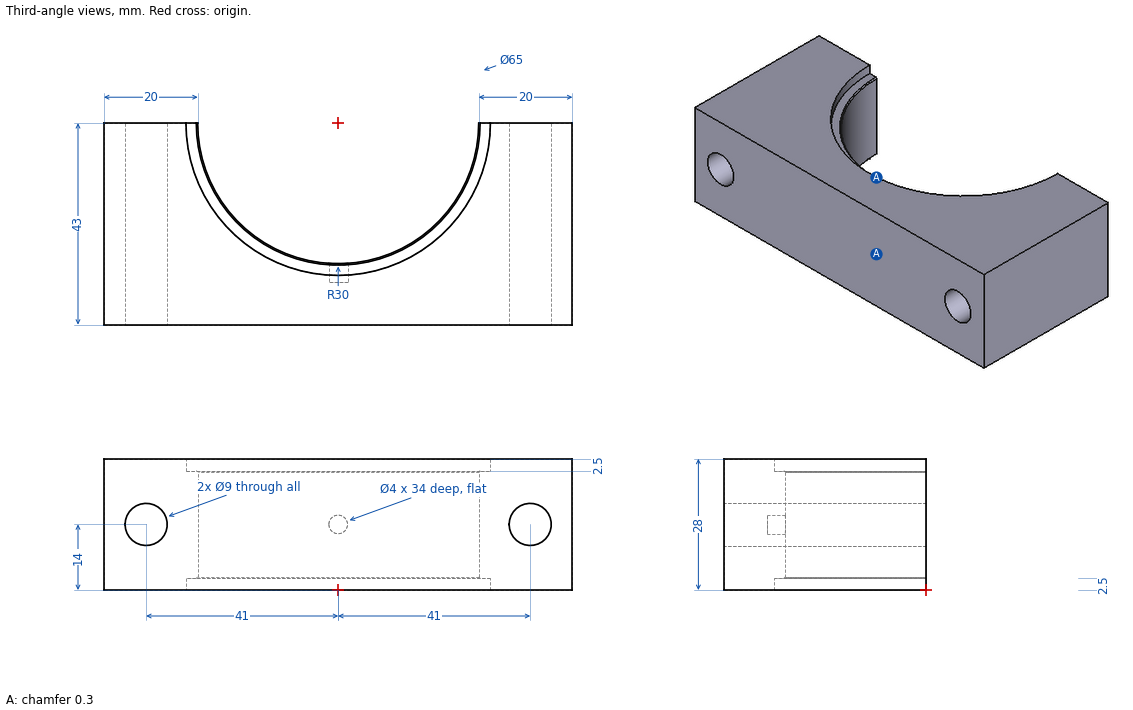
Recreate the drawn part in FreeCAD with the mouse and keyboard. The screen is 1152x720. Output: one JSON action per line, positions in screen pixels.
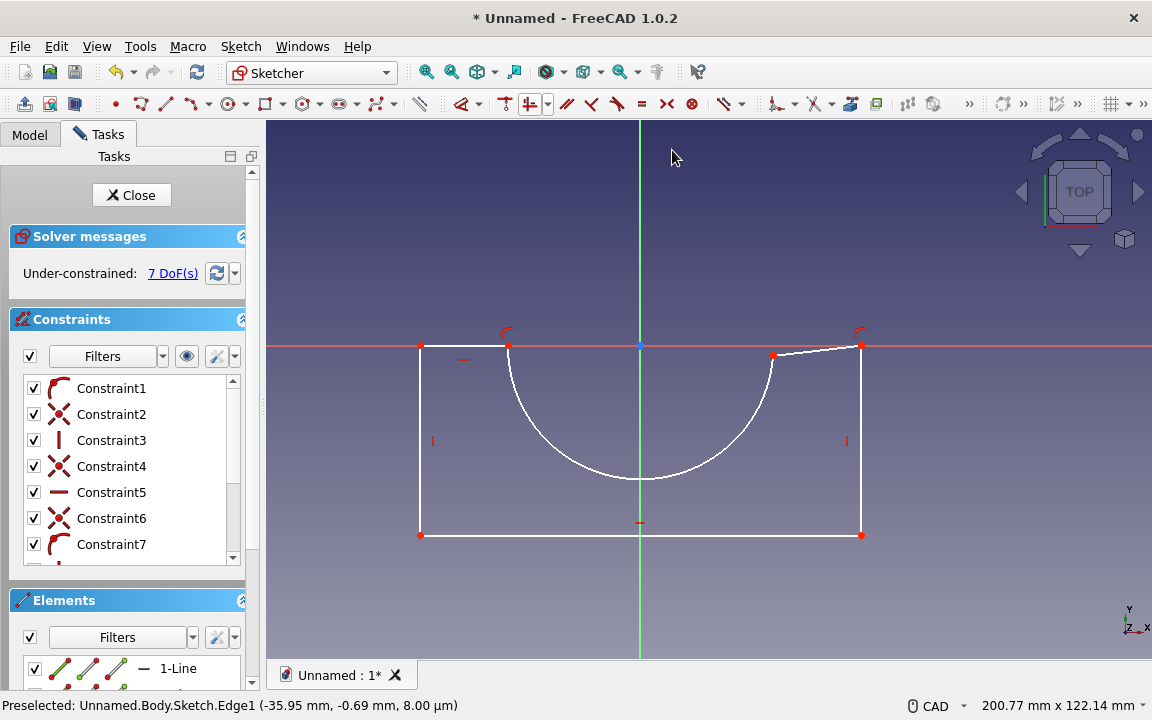
{"action": "left_click", "coordinate": [835, 349]}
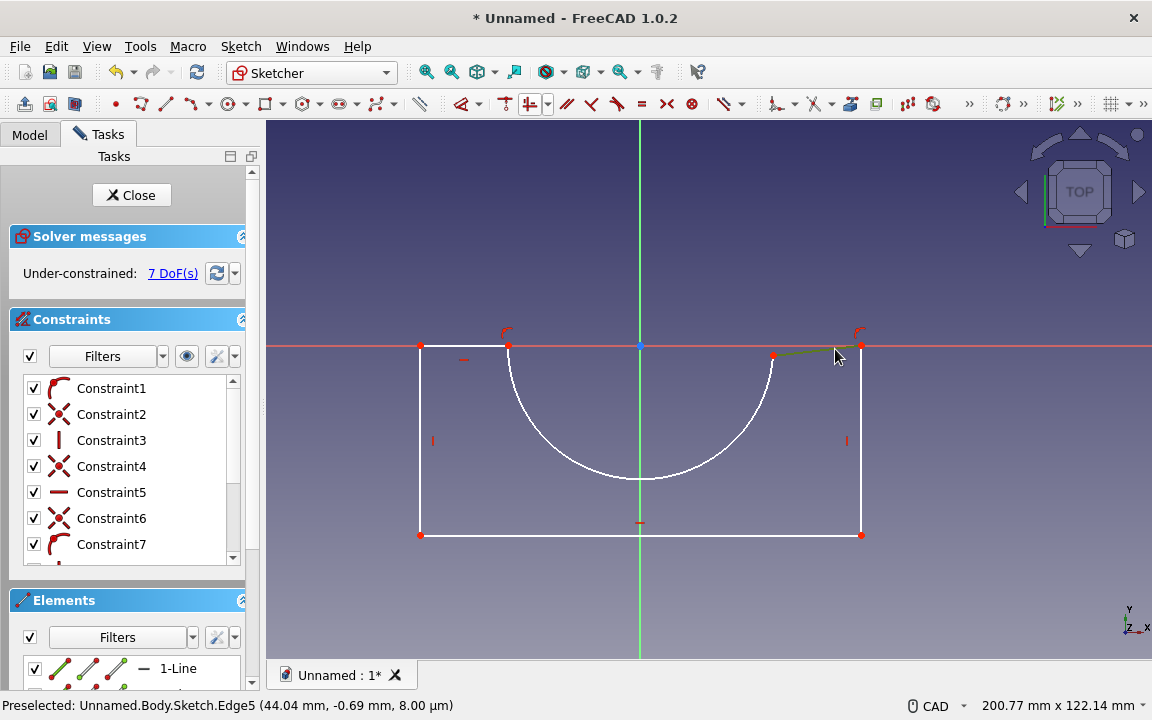
{"action": "left_click", "coordinate": [548, 104]}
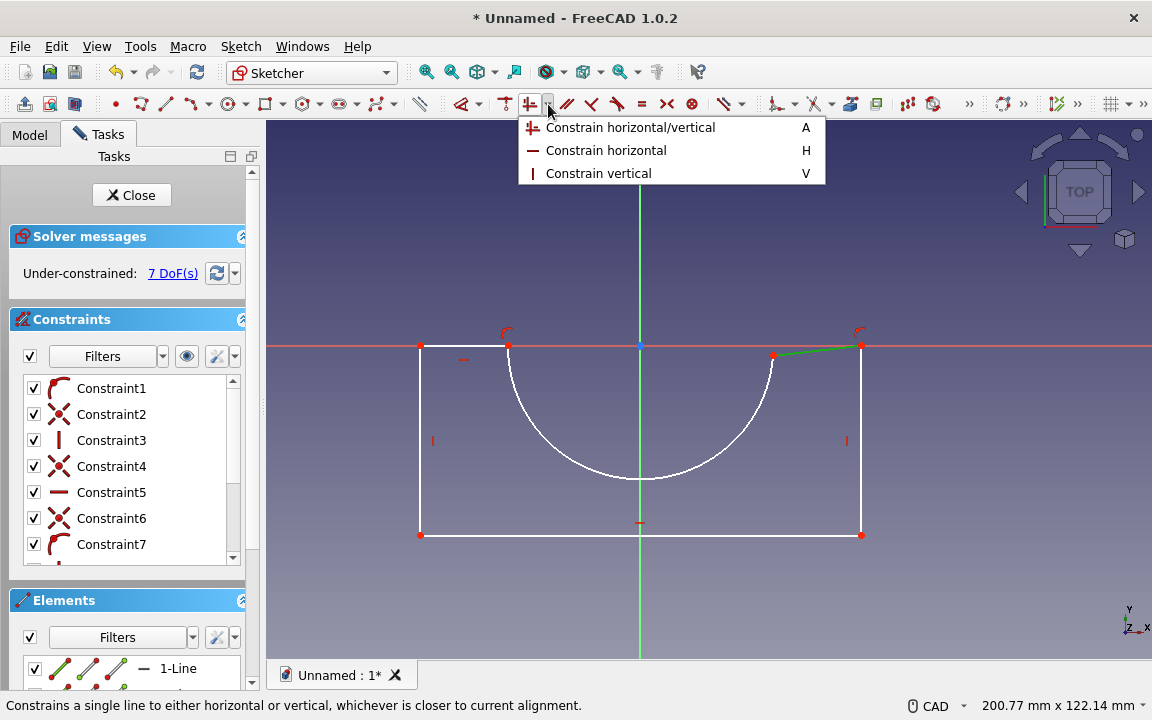
{"action": "left_click", "coordinate": [672, 150]}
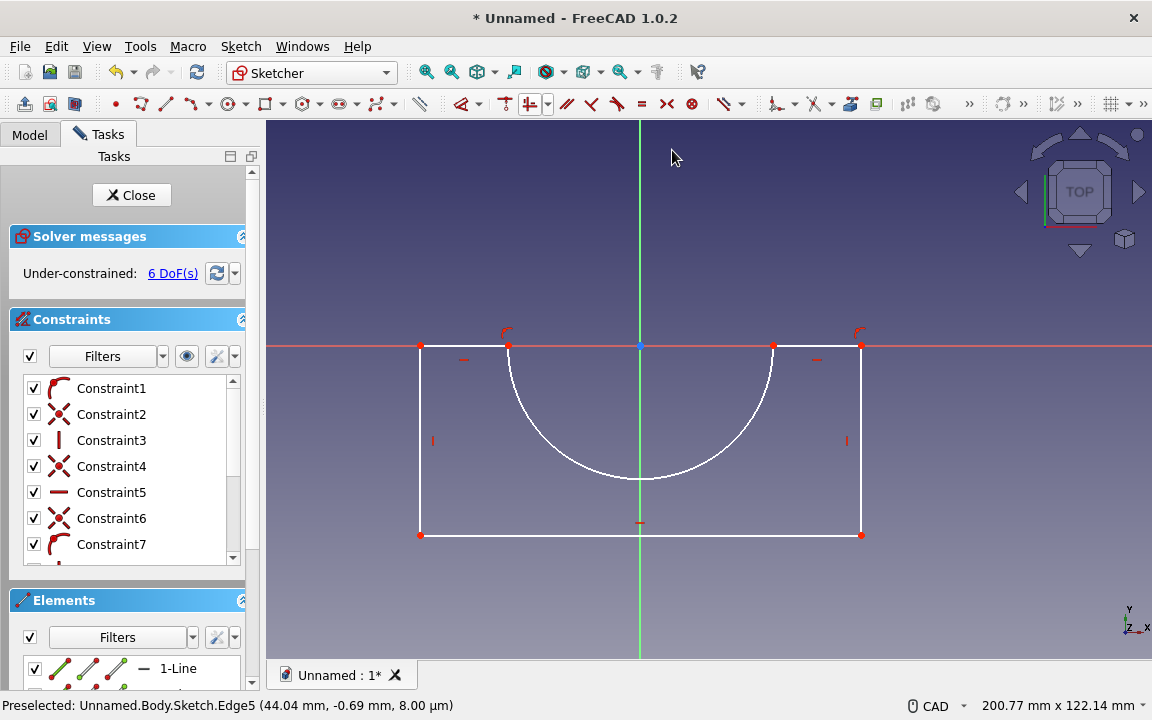
{"action": "left_click_drag", "start_coordinate": [630, 336], "coordinate": [651, 357]}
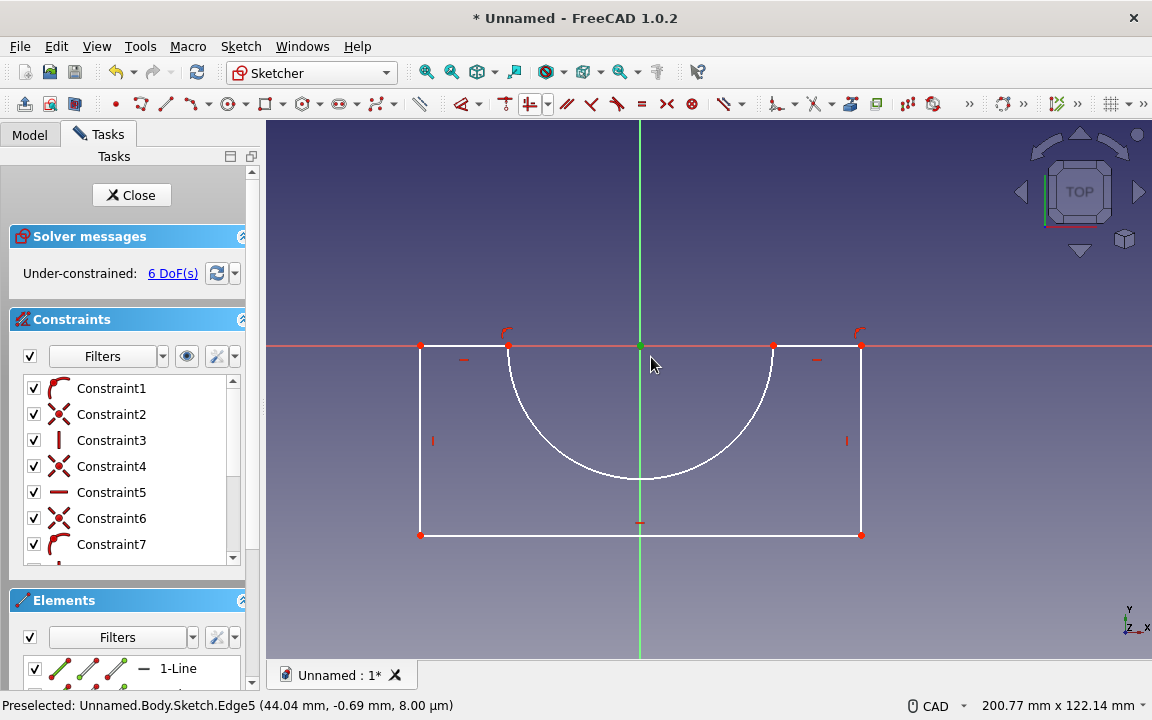
{"action": "left_click", "coordinate": [505, 104]}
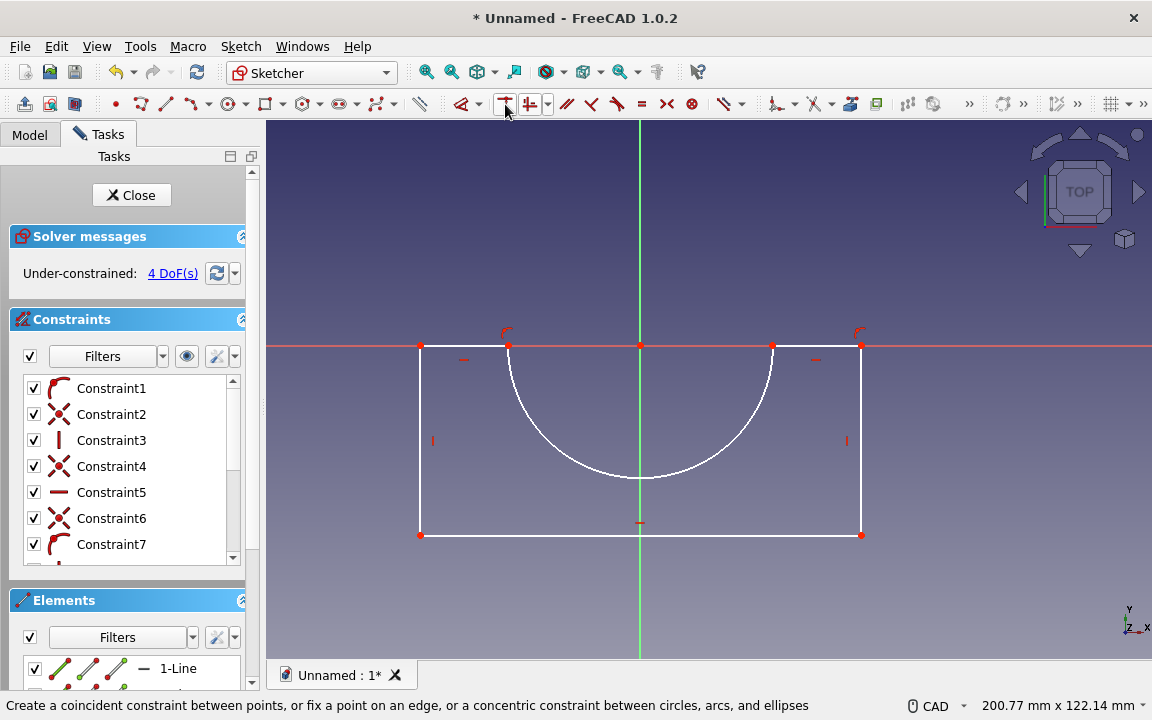
{"action": "left_click", "coordinate": [460, 104]}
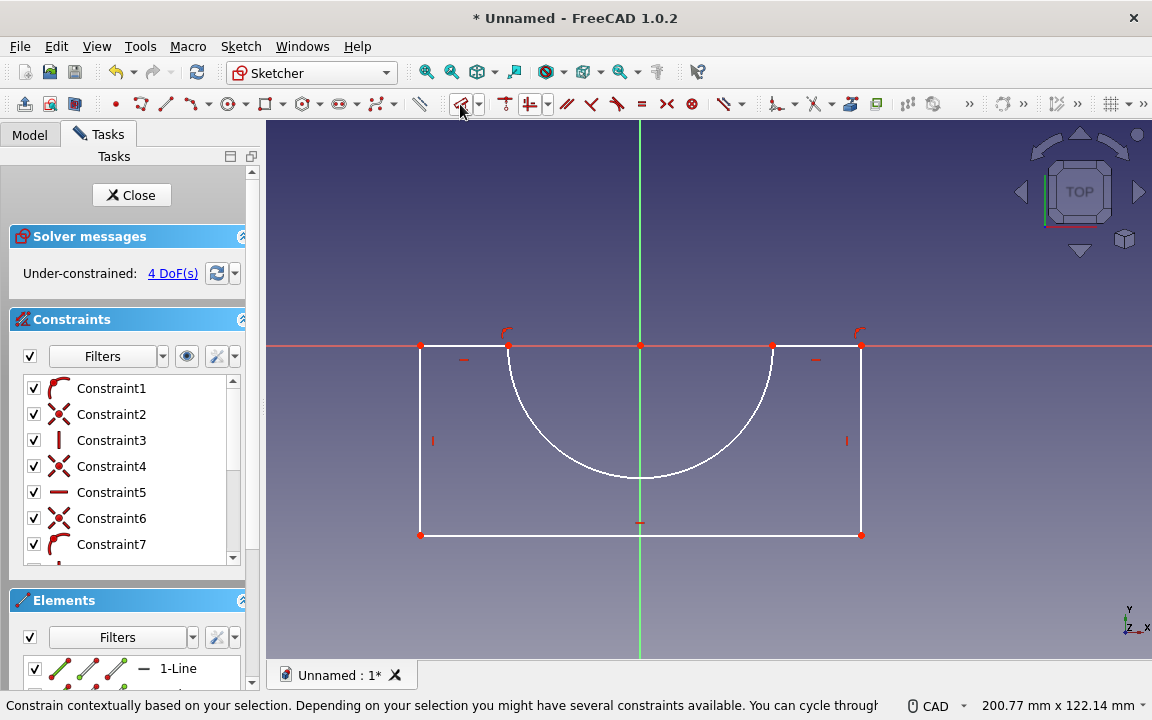
{"action": "left_click", "coordinate": [563, 453]}
{"action": "left_click", "coordinate": [544, 479]}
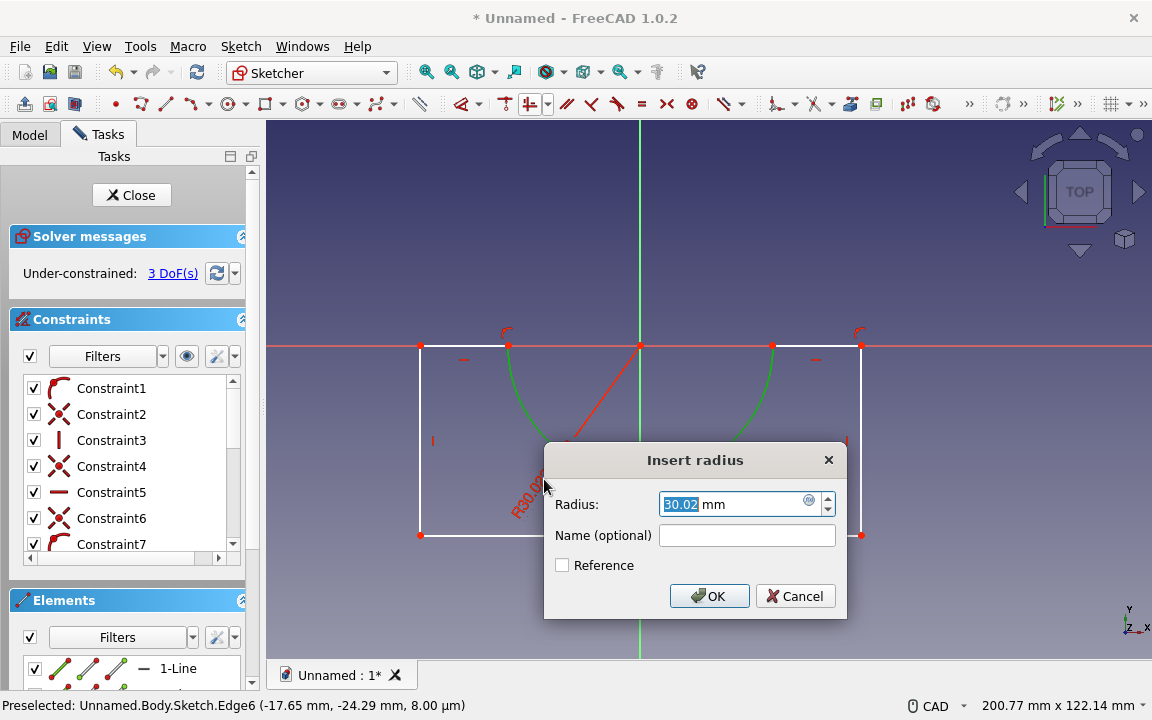
{"action": "type", "text": "30"}
{"action": "key", "text": "Return"}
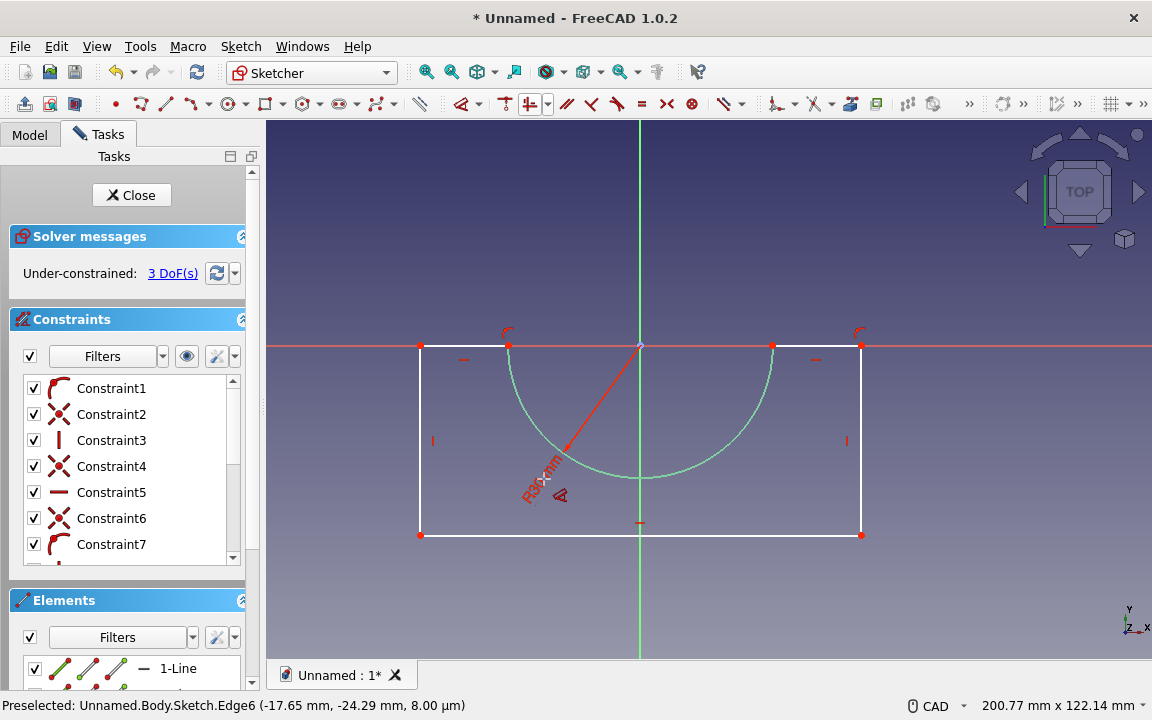
{"action": "left_click", "coordinate": [482, 346]}
{"action": "left_click", "coordinate": [464, 312]}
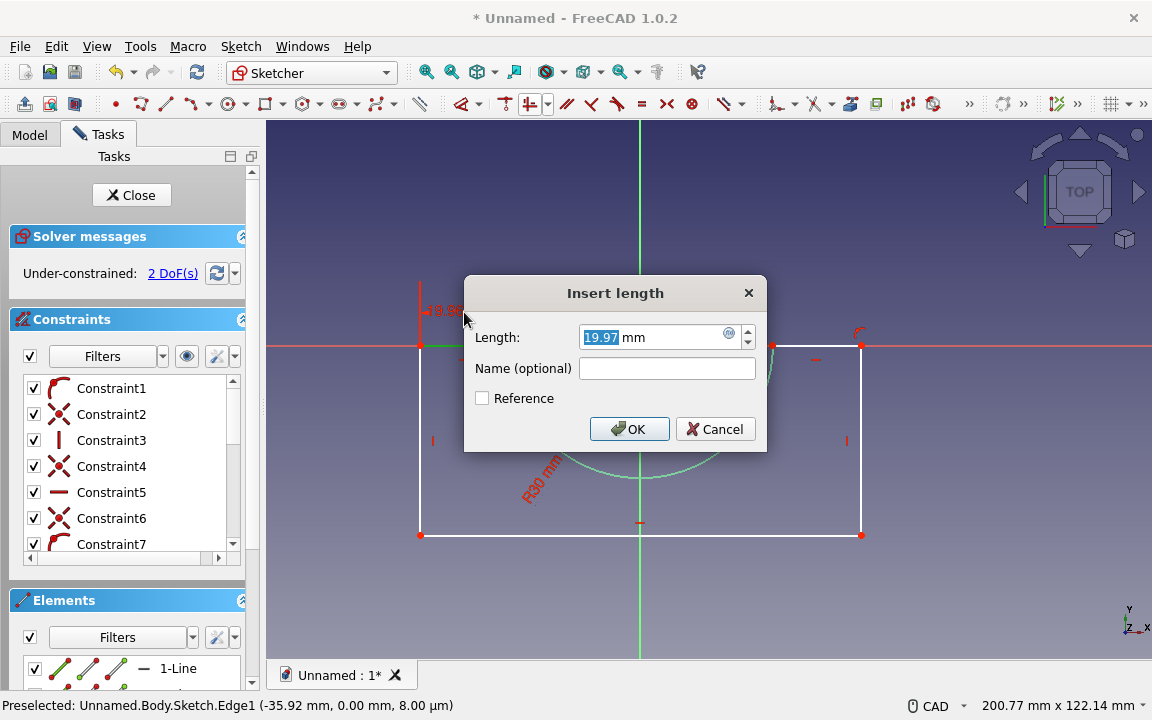
{"action": "type", "text": "20"}
{"action": "key", "text": "Return"}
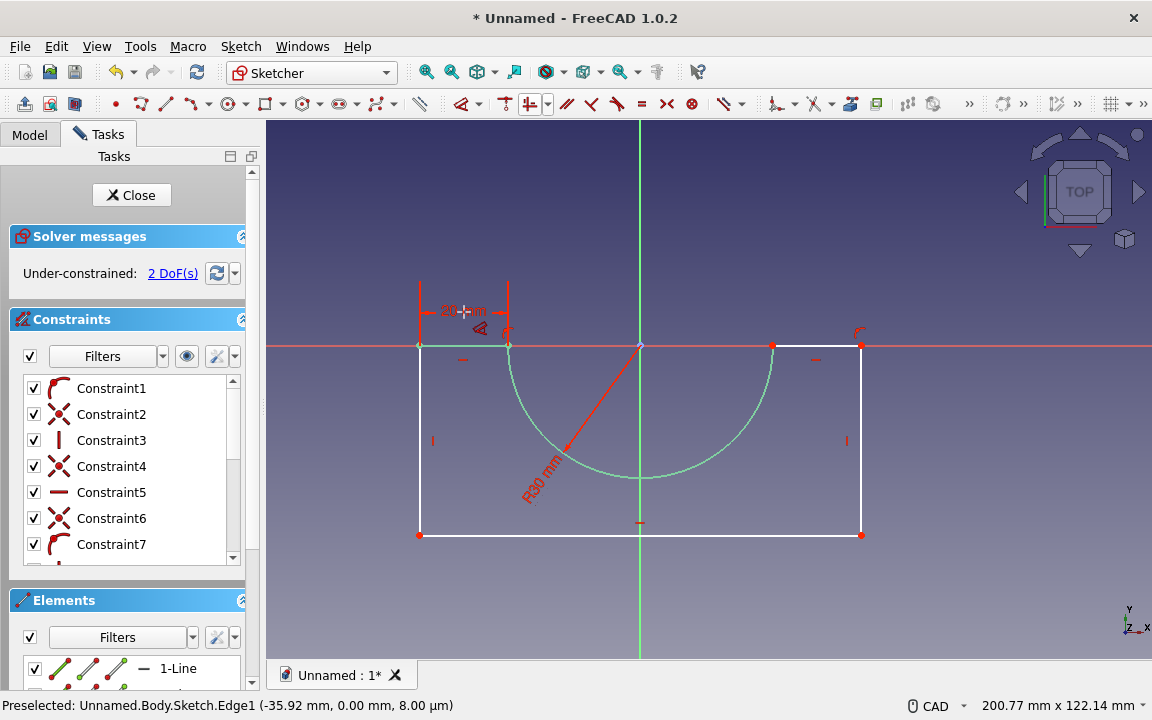
{"action": "left_click", "coordinate": [420, 403]}
{"action": "left_click", "coordinate": [386, 441]}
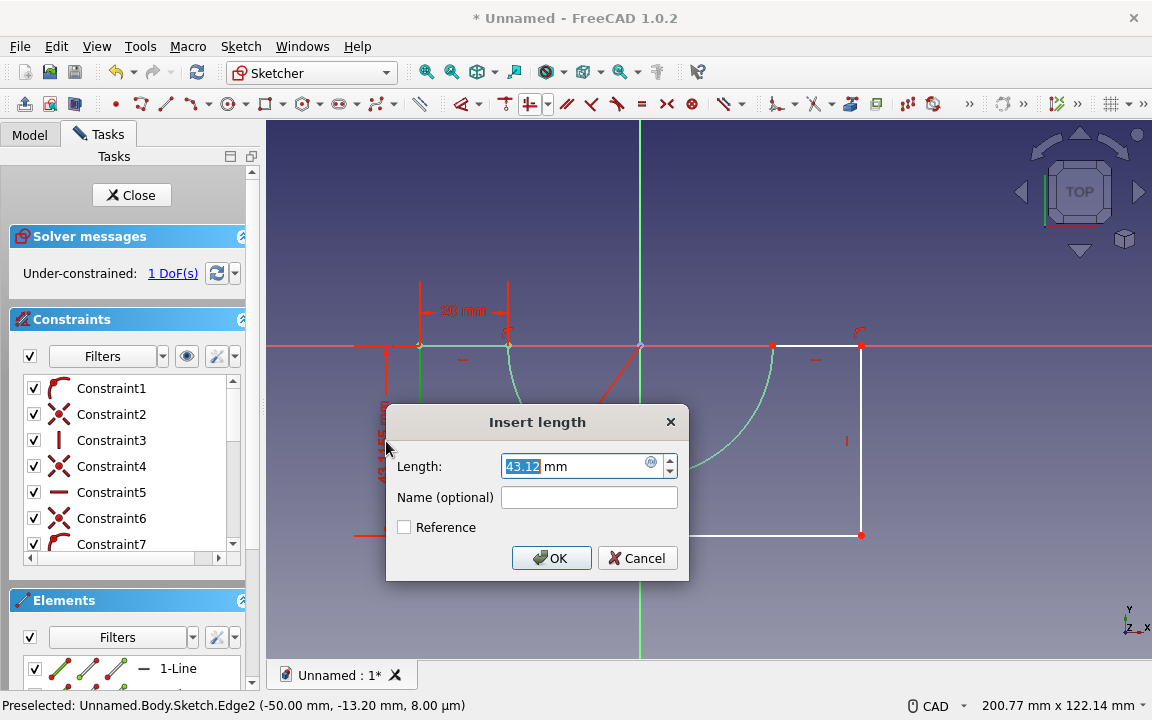
{"action": "type", "text": "43"}
{"action": "key", "text": "Return"}